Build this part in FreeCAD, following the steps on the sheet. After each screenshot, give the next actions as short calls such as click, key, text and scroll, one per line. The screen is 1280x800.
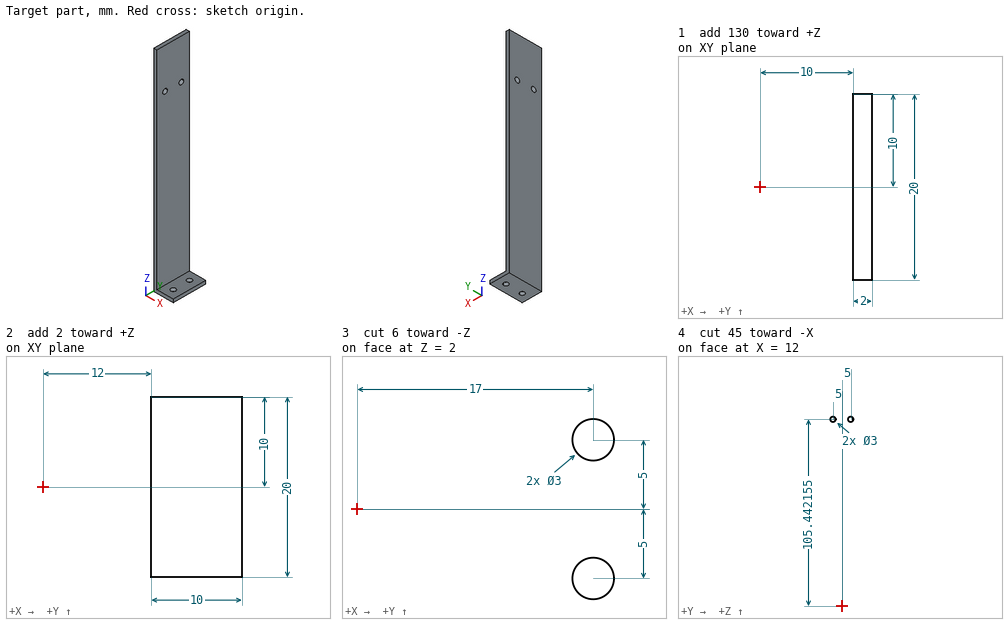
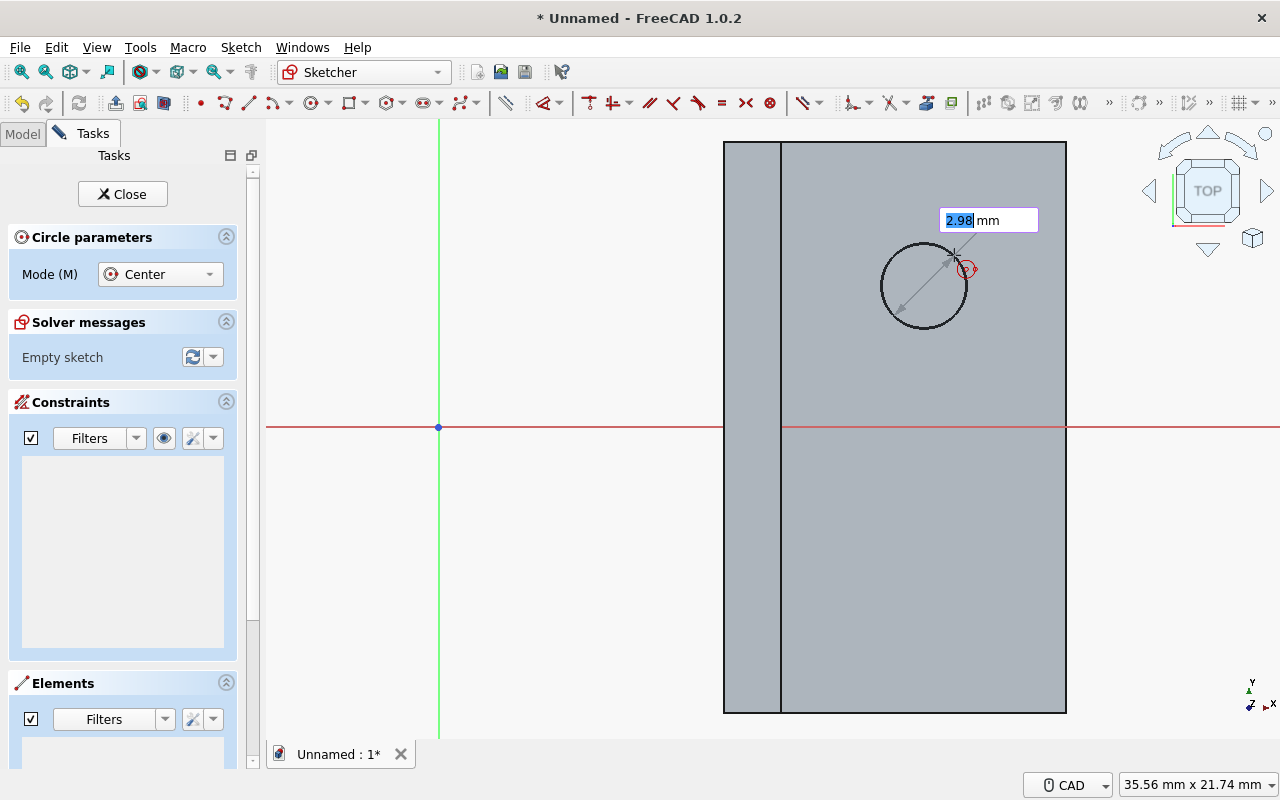
text(3)
key(Return)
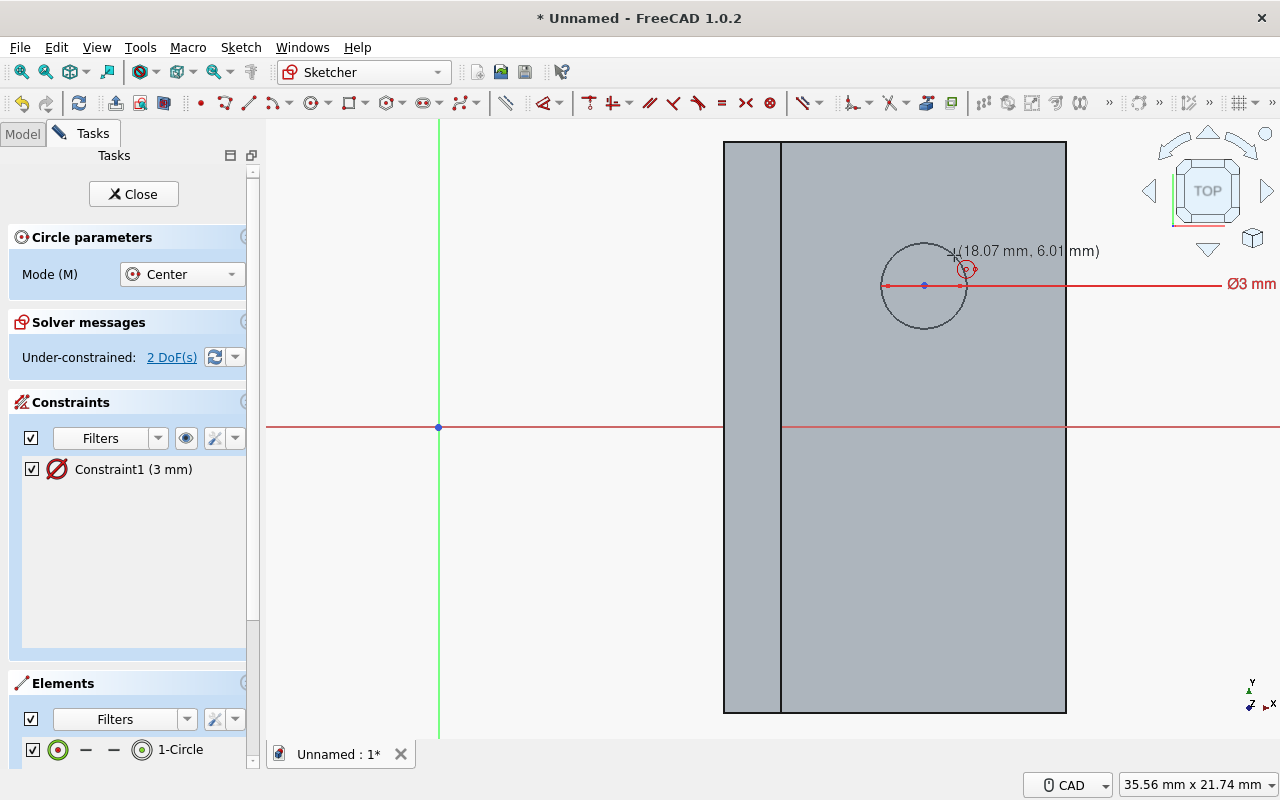
click(924, 570)
move(954, 540)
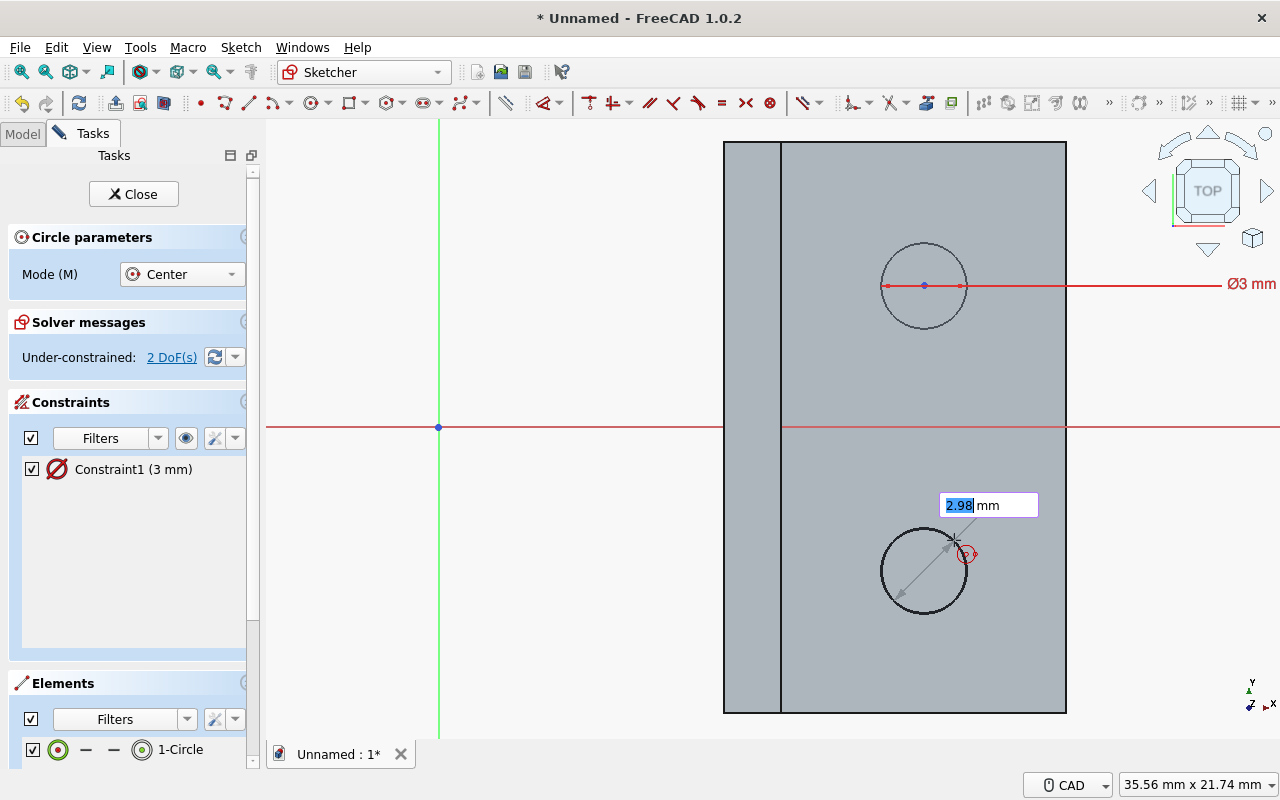
text(3)
key(Return)
key(Escape)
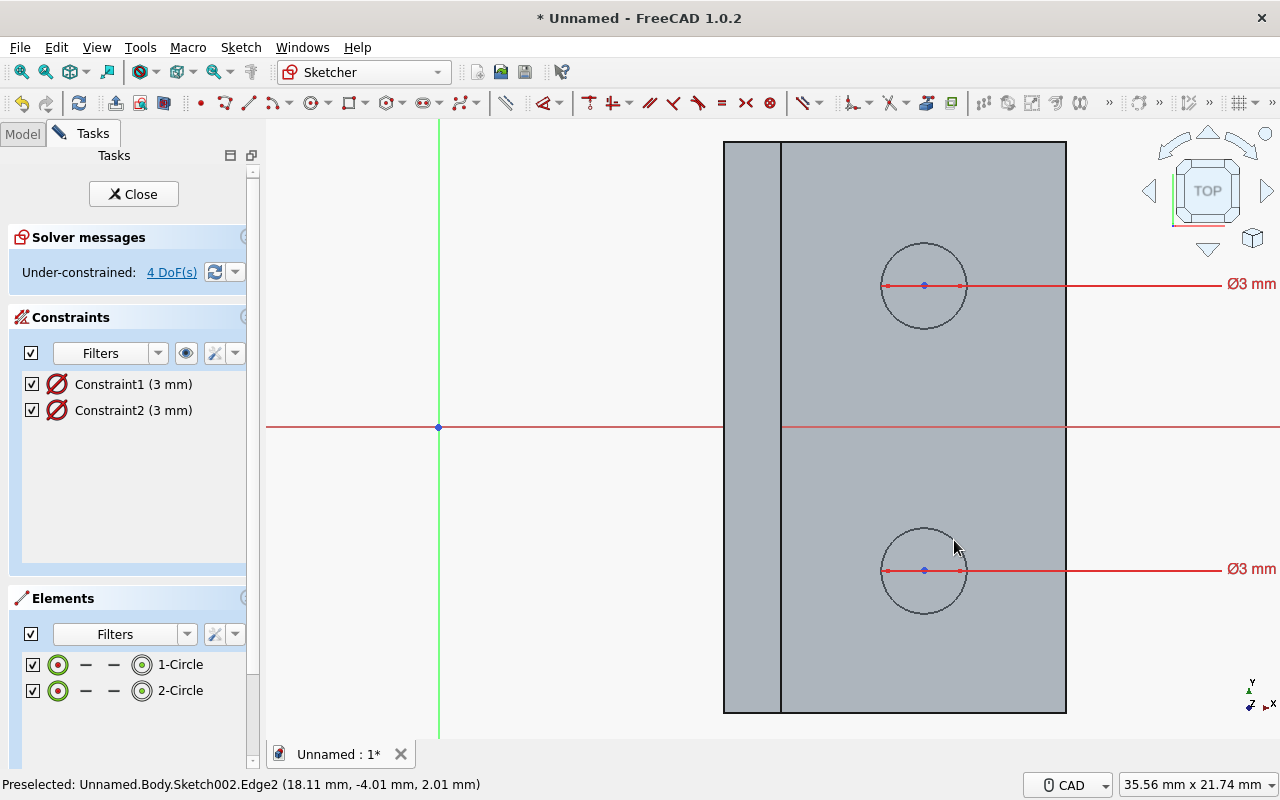
click(924, 286)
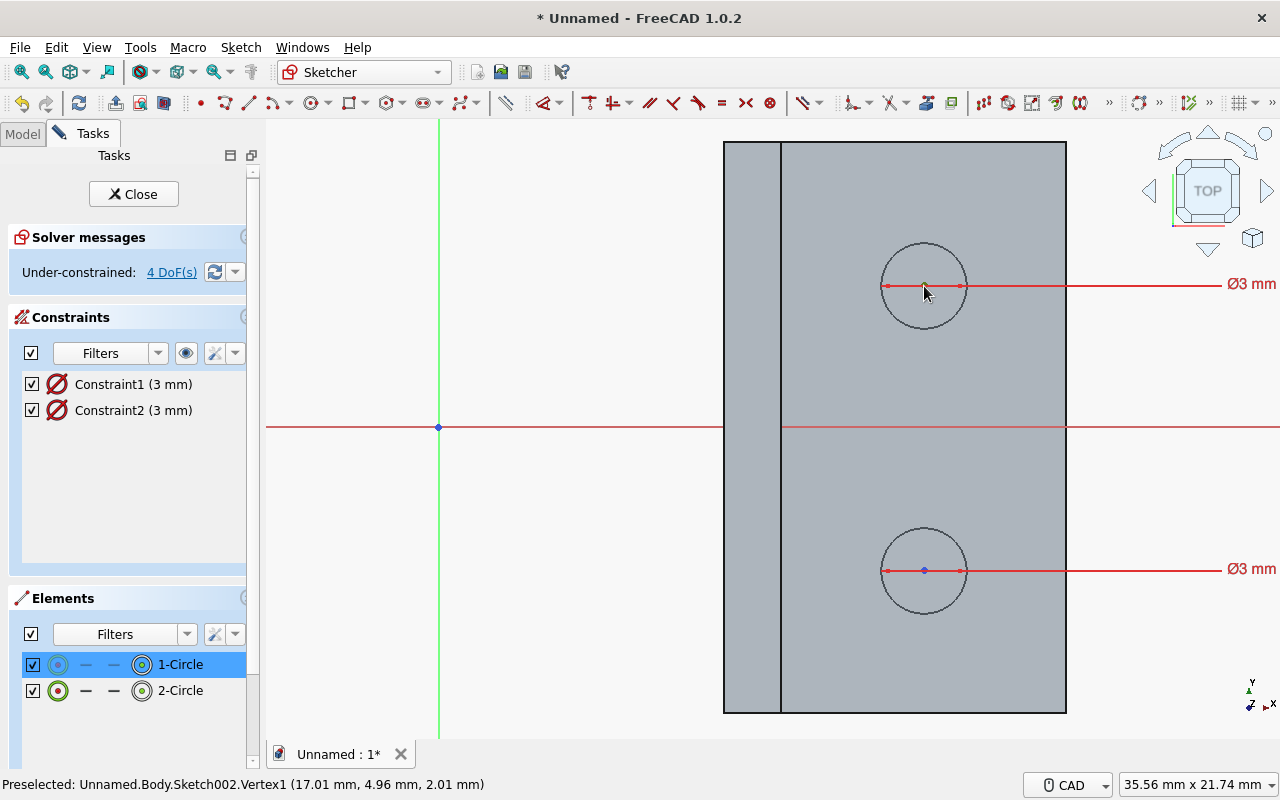
click(924, 571)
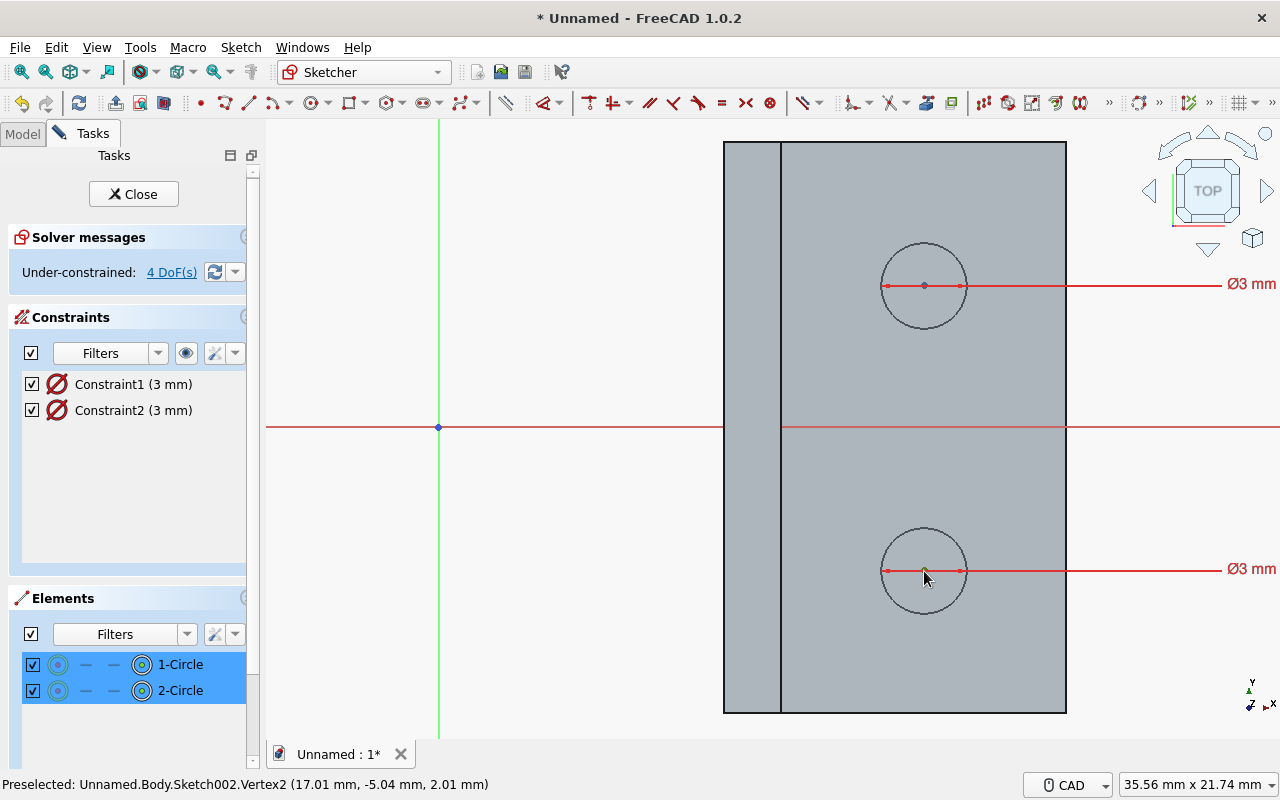
key(v)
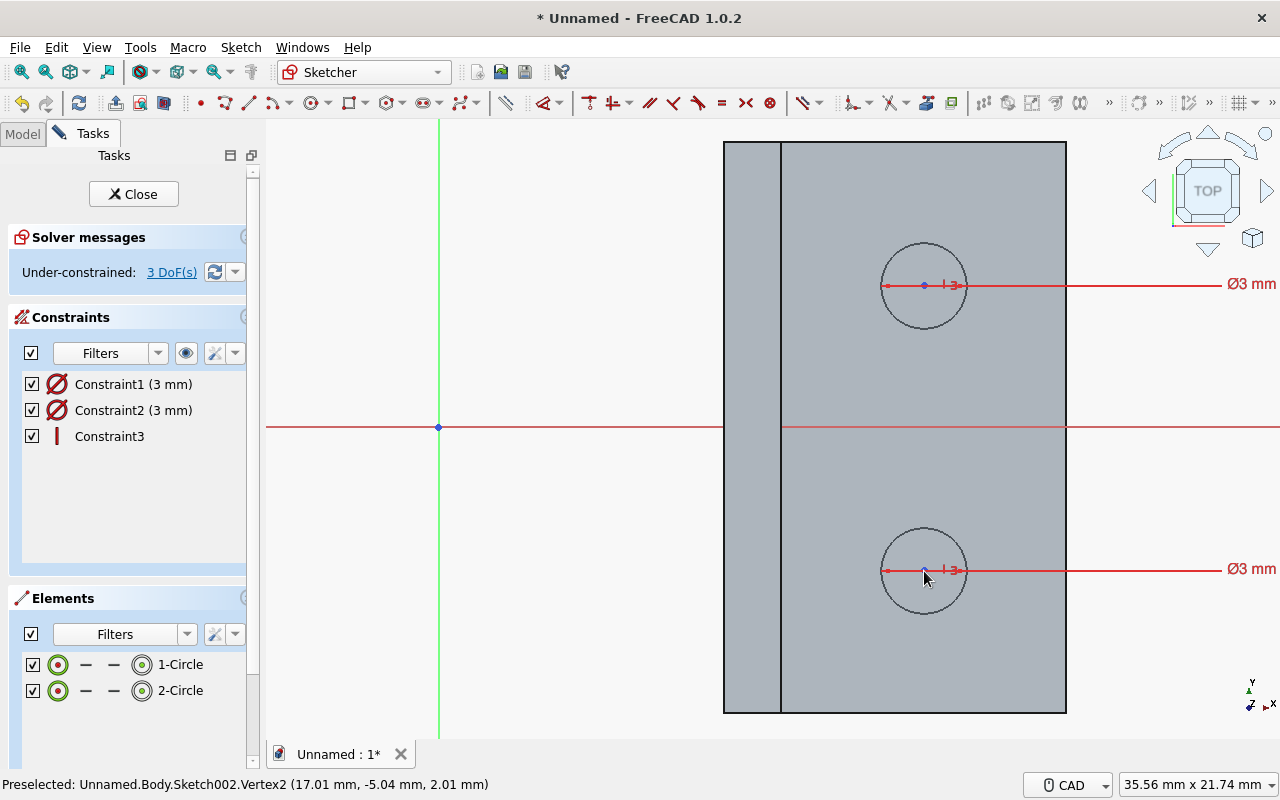
key(d)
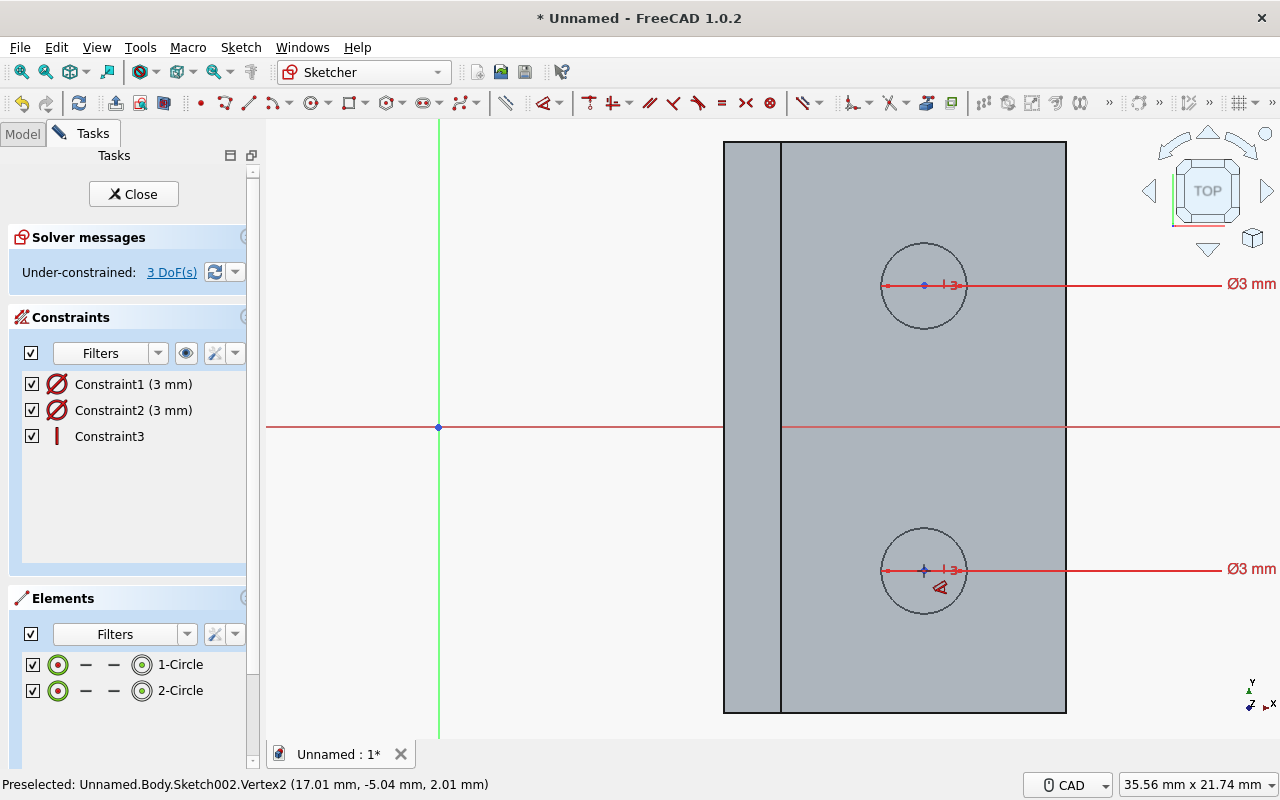
click(924, 286)
click(405, 357)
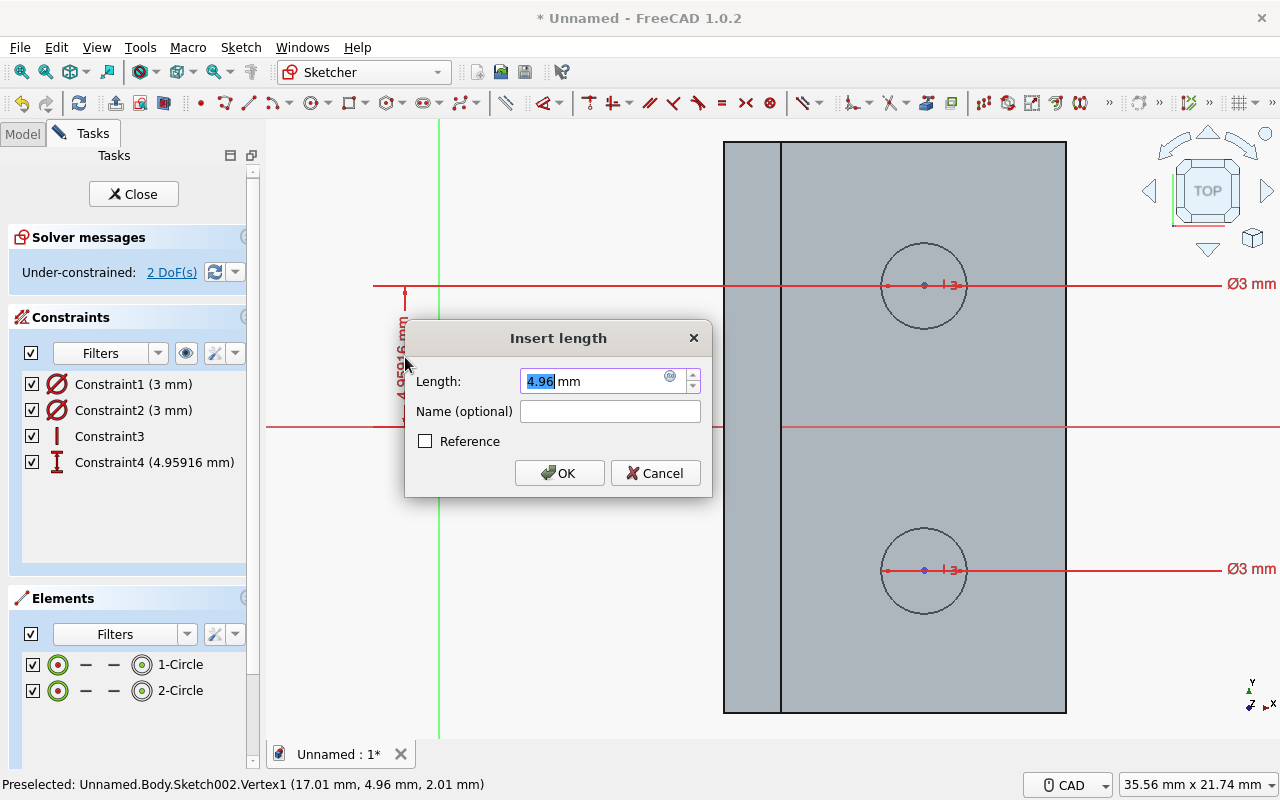
text(5)
key(Return)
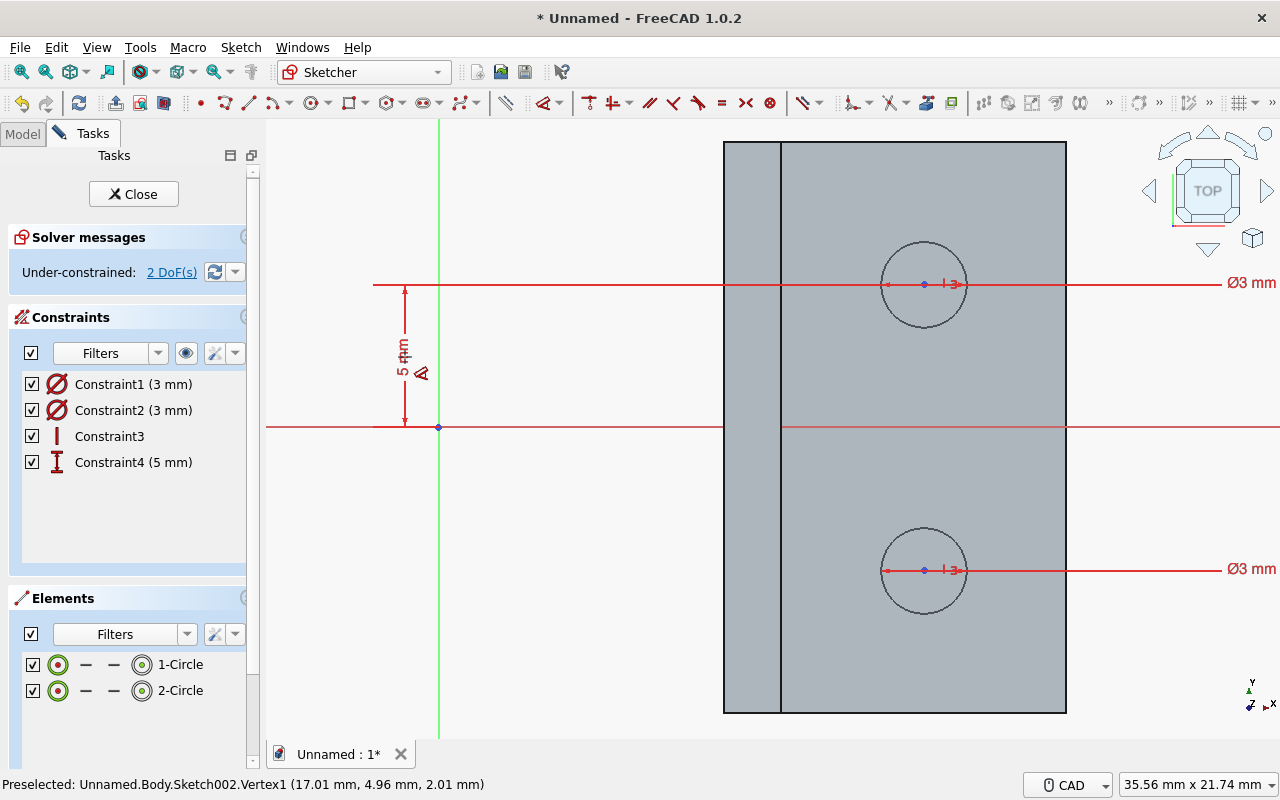
click(924, 571)
click(405, 499)